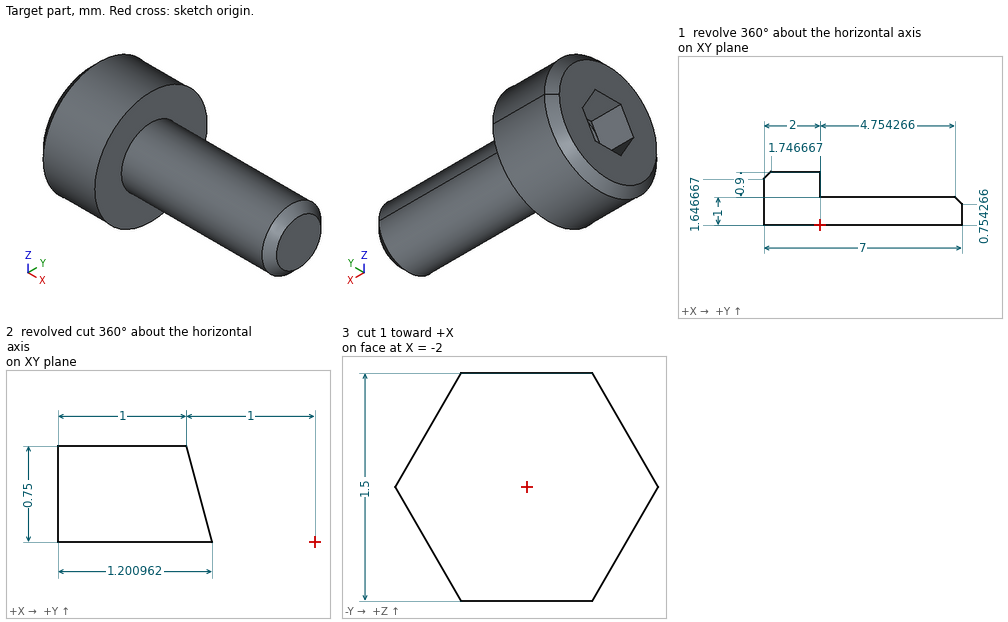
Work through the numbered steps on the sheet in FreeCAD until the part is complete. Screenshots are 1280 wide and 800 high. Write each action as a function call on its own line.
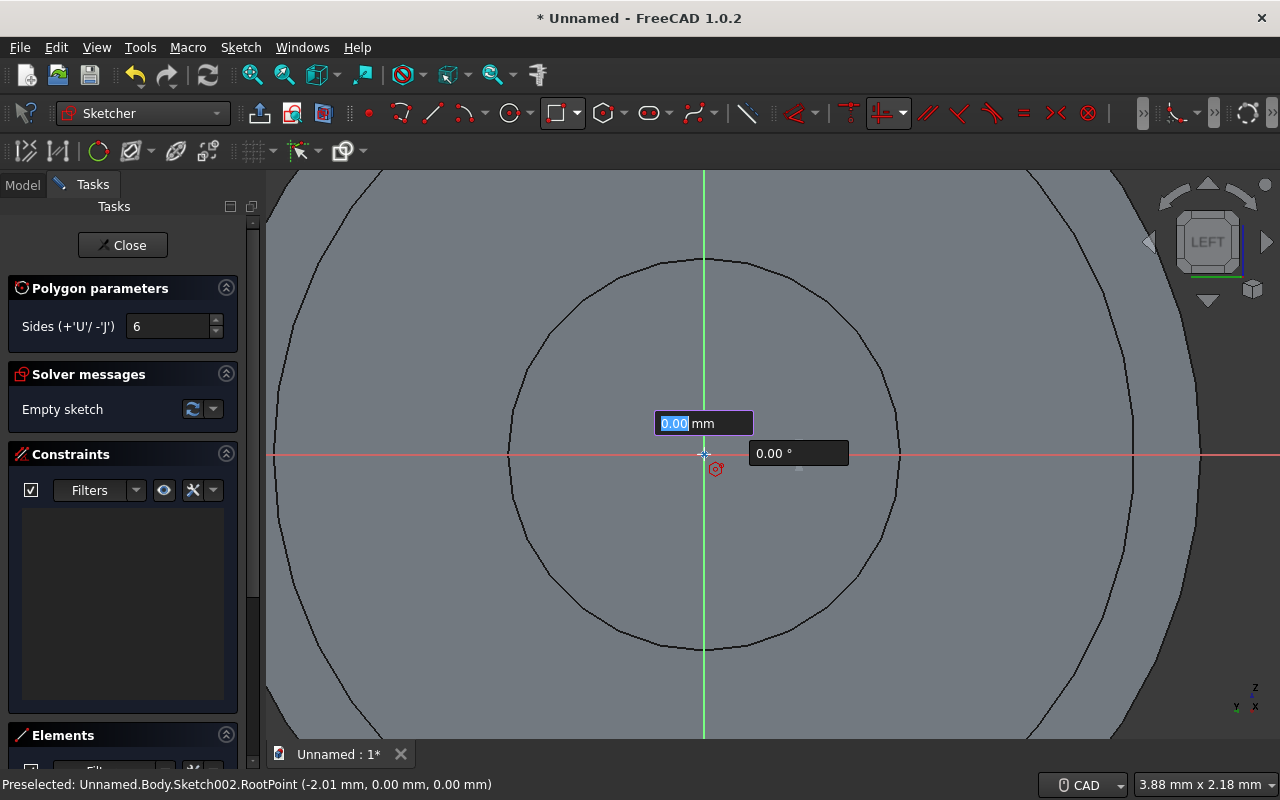
click(931, 454)
right_click(931, 454)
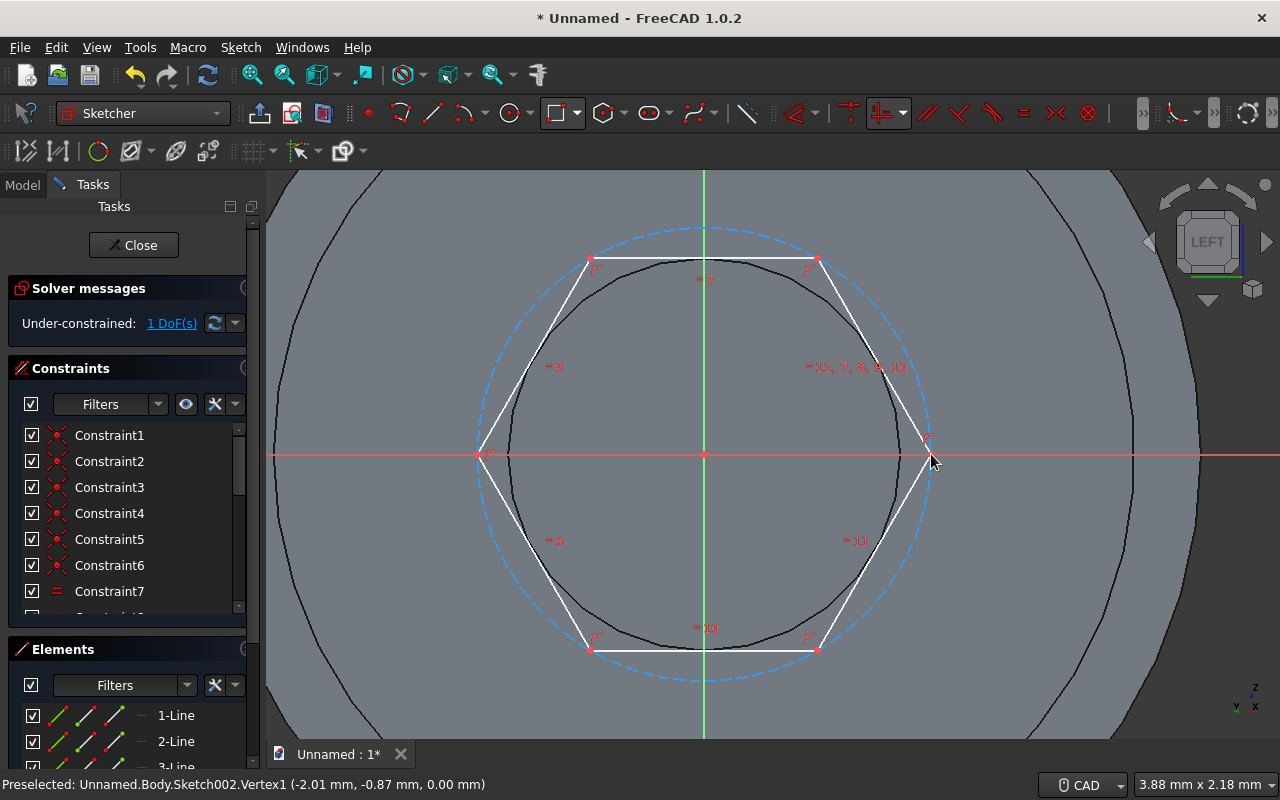
click(794, 114)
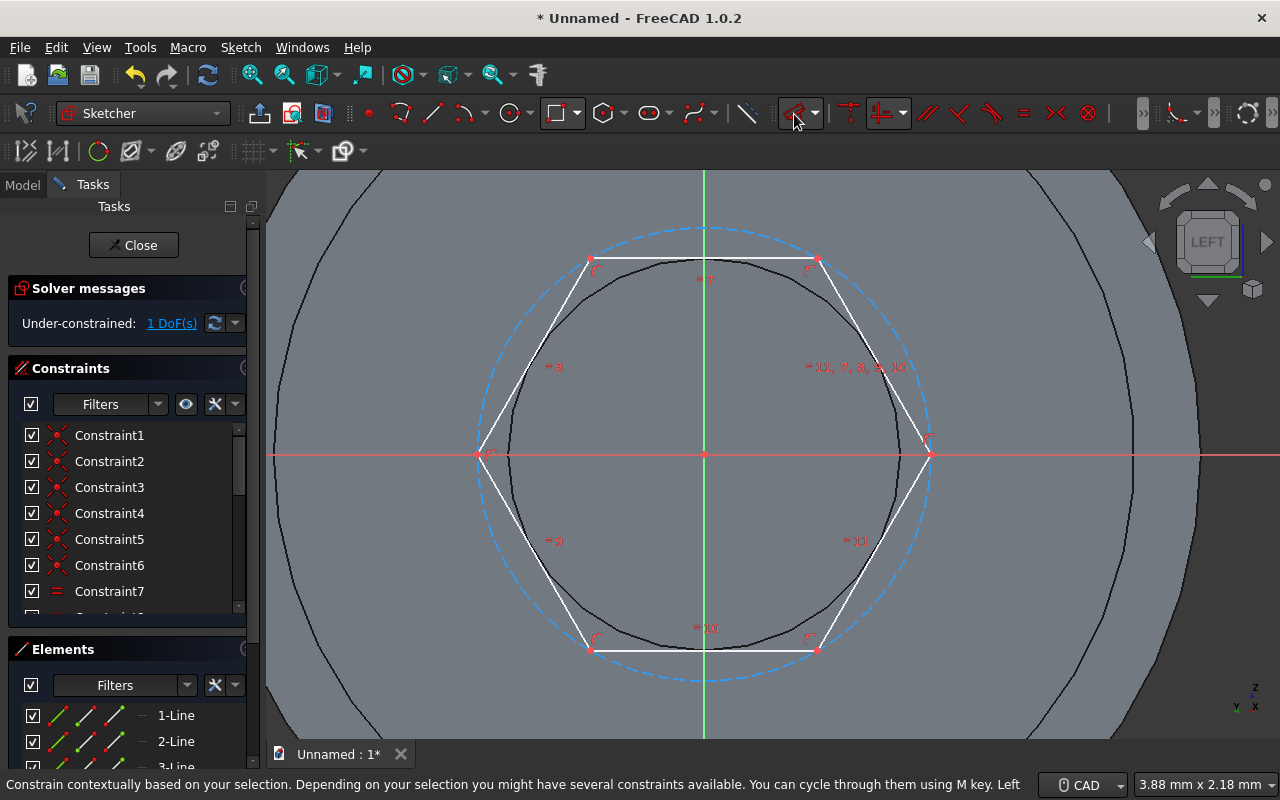
click(591, 651)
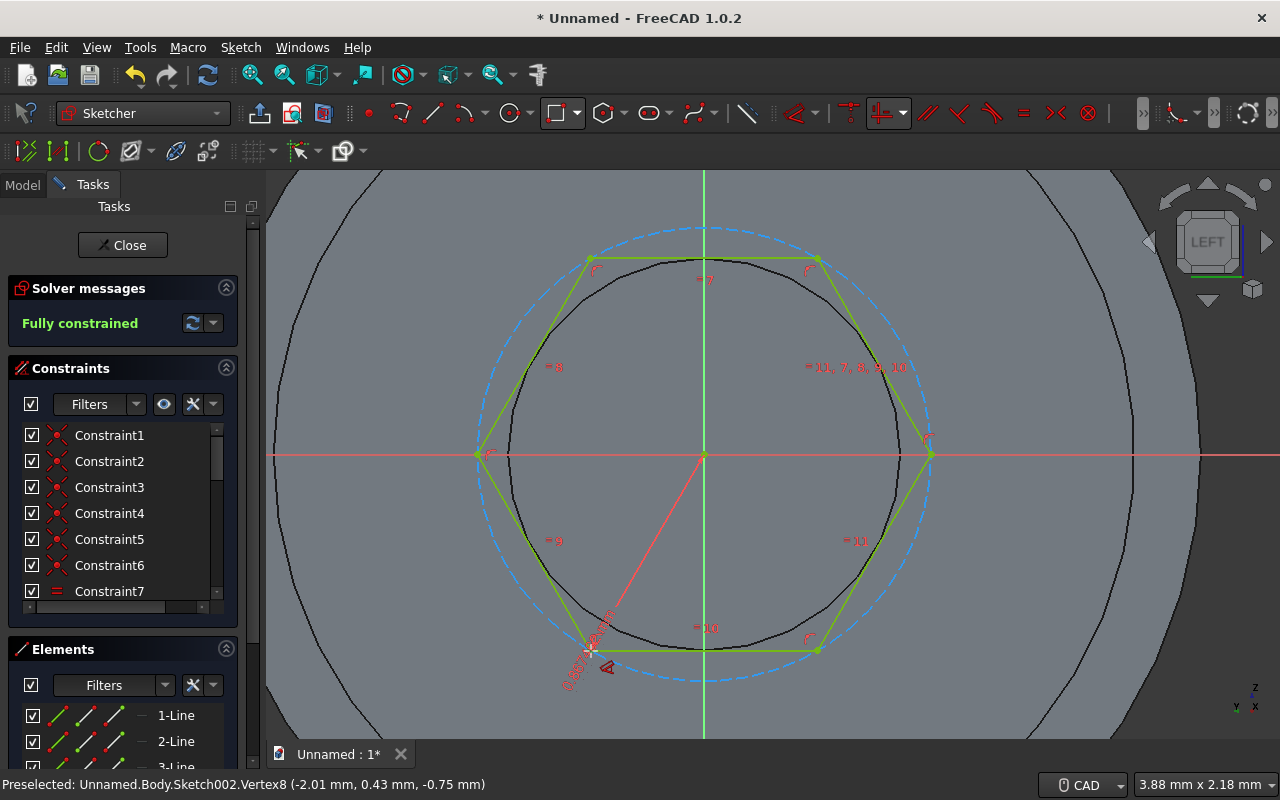
click(818, 258)
click(557, 364)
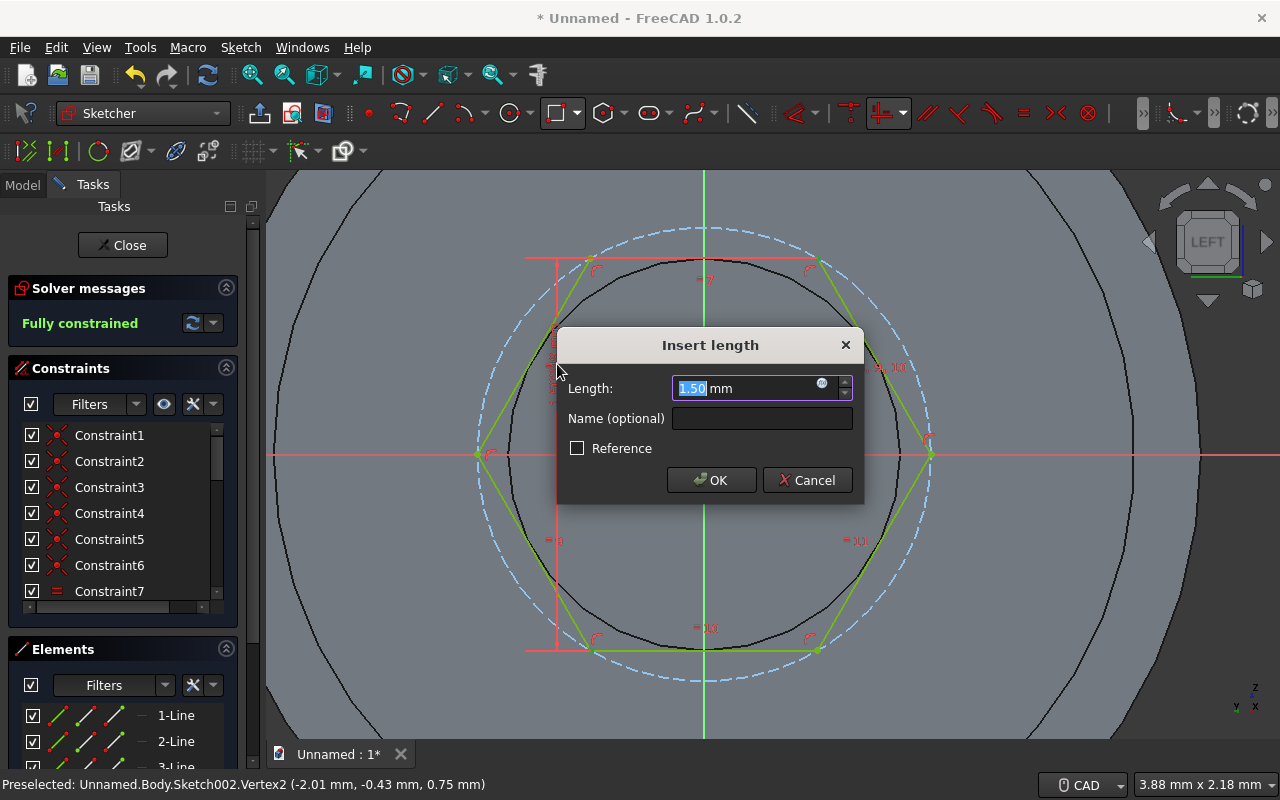
text(1.5)
key(Return)
key(Escape)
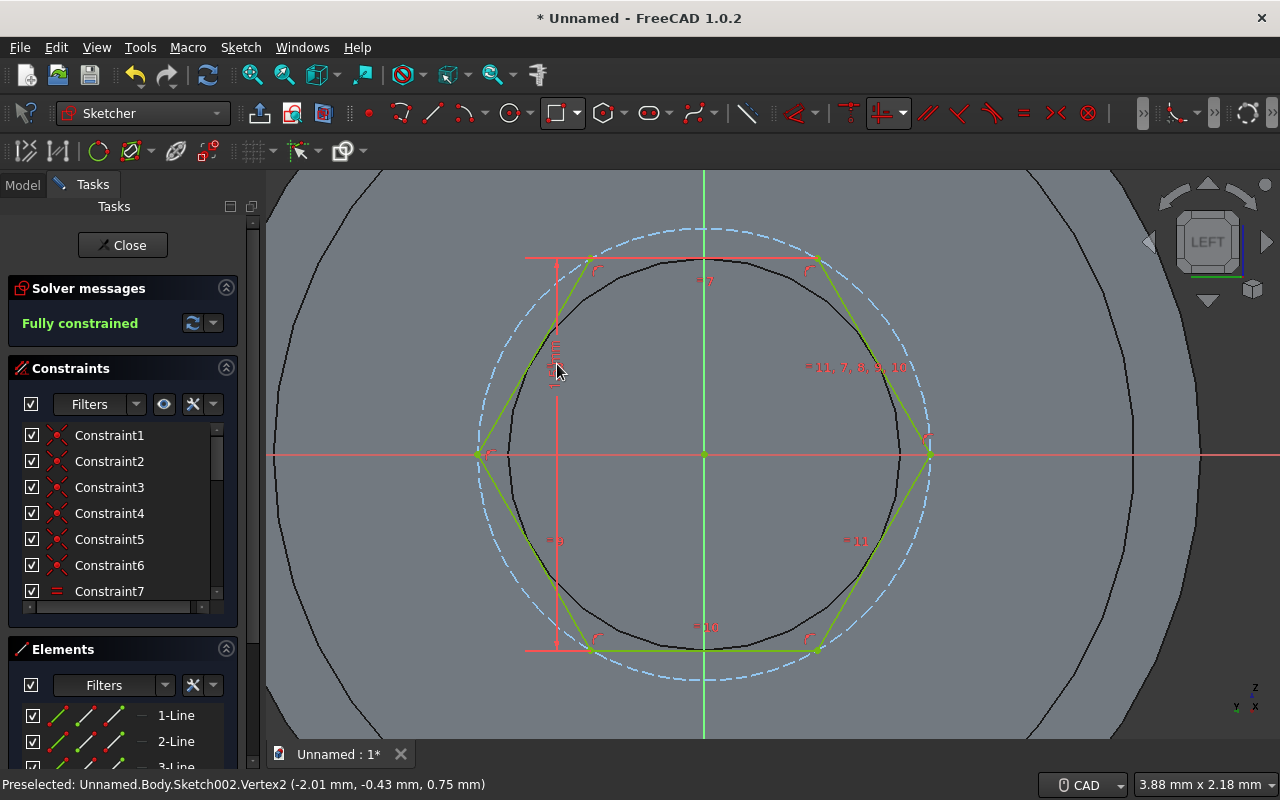
click(123, 245)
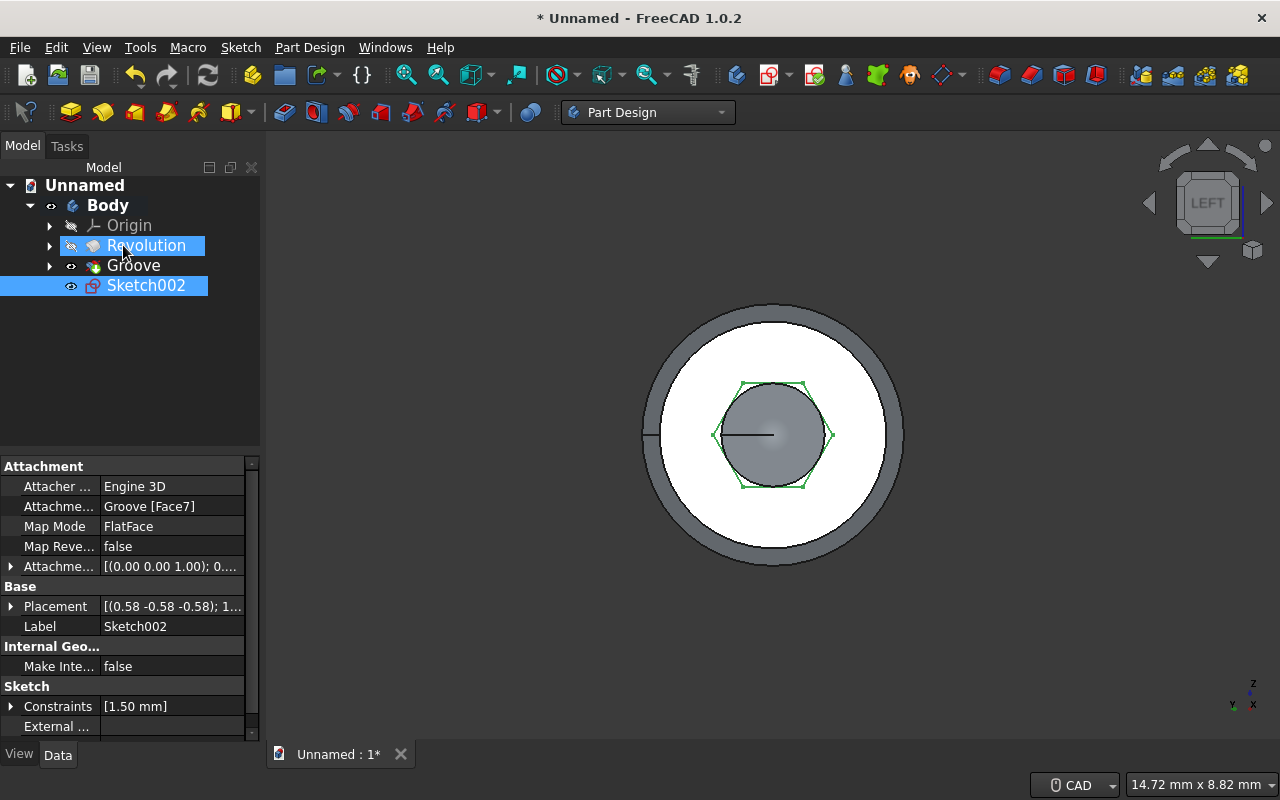
click(286, 112)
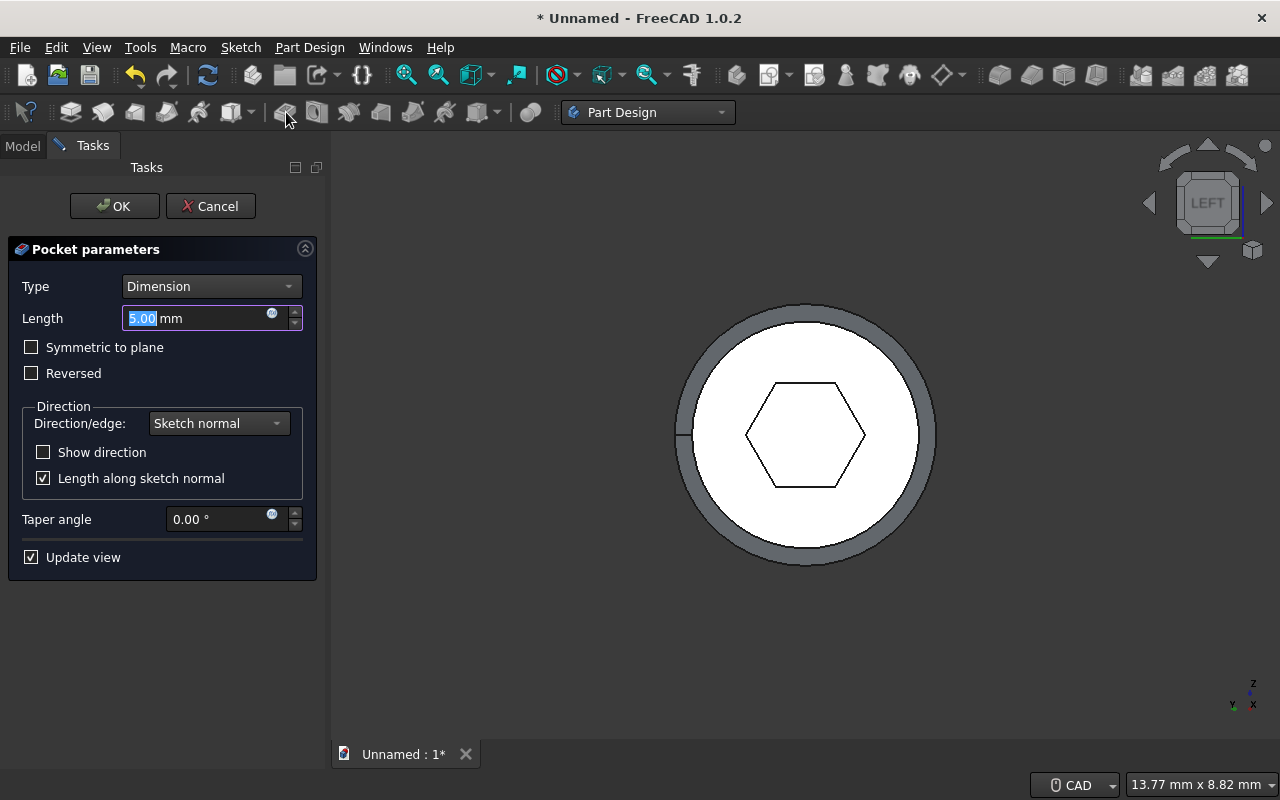
text(1)
key(Tab)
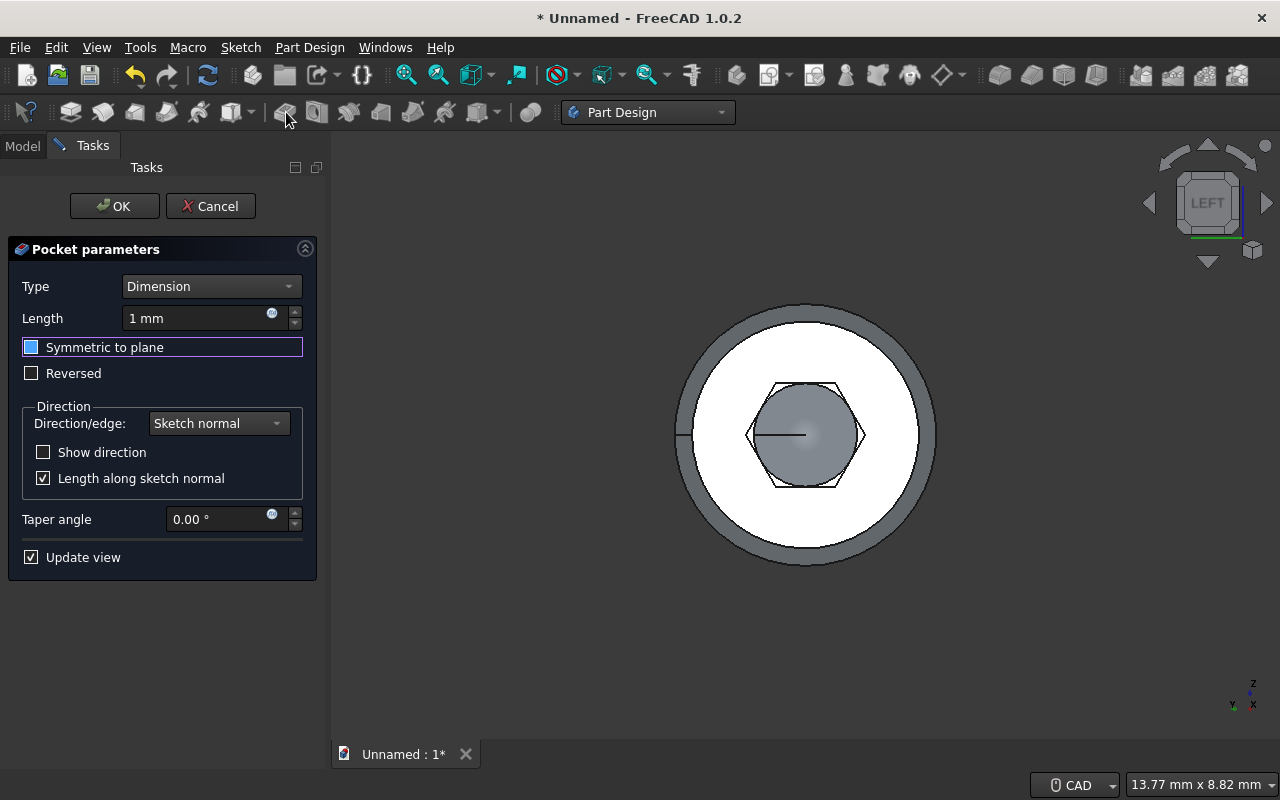
click(115, 206)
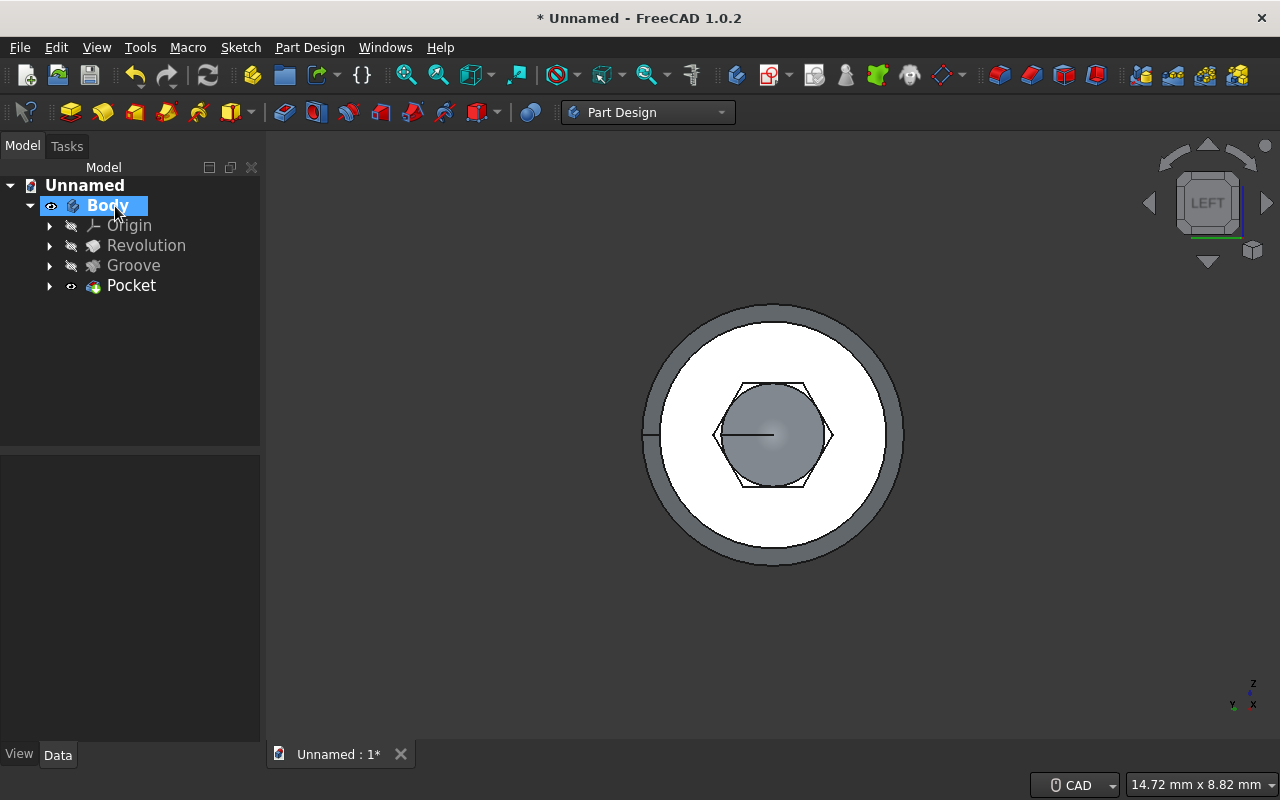
key(0)